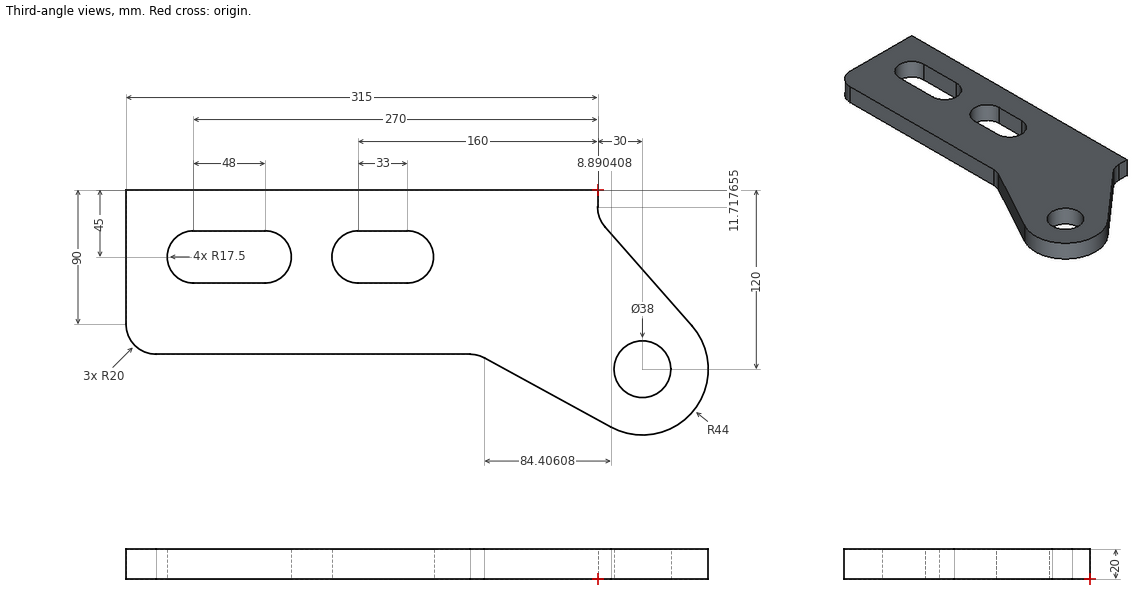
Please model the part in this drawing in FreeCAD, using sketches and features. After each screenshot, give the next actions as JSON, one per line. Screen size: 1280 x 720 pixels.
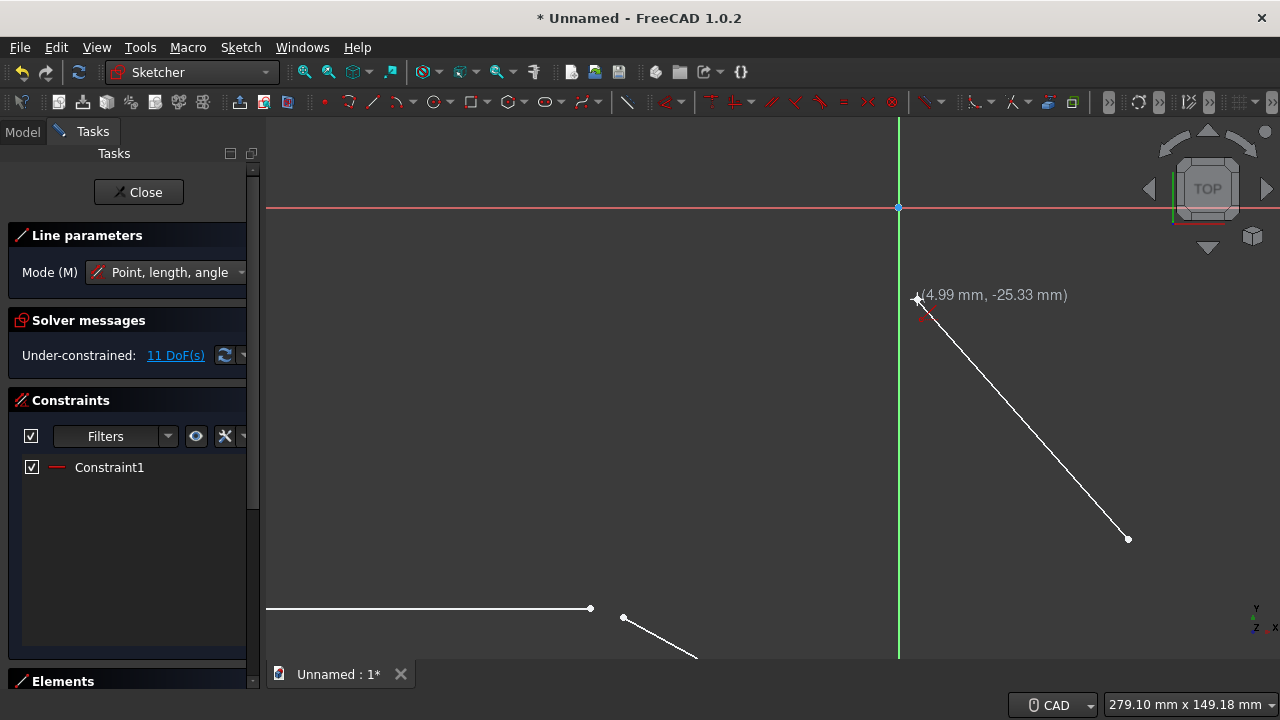
{"action": "left_click", "coordinate": [350, 102]}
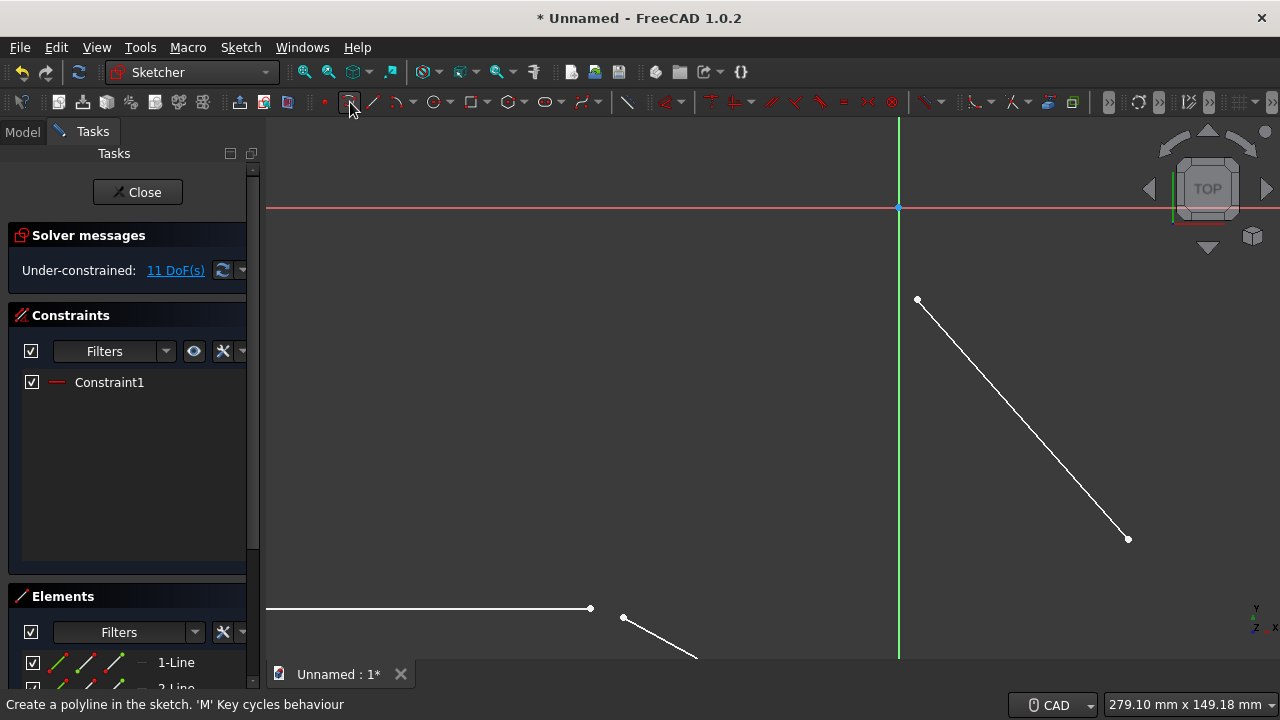
{"action": "left_click", "coordinate": [899, 251]}
{"action": "left_click", "coordinate": [899, 208]}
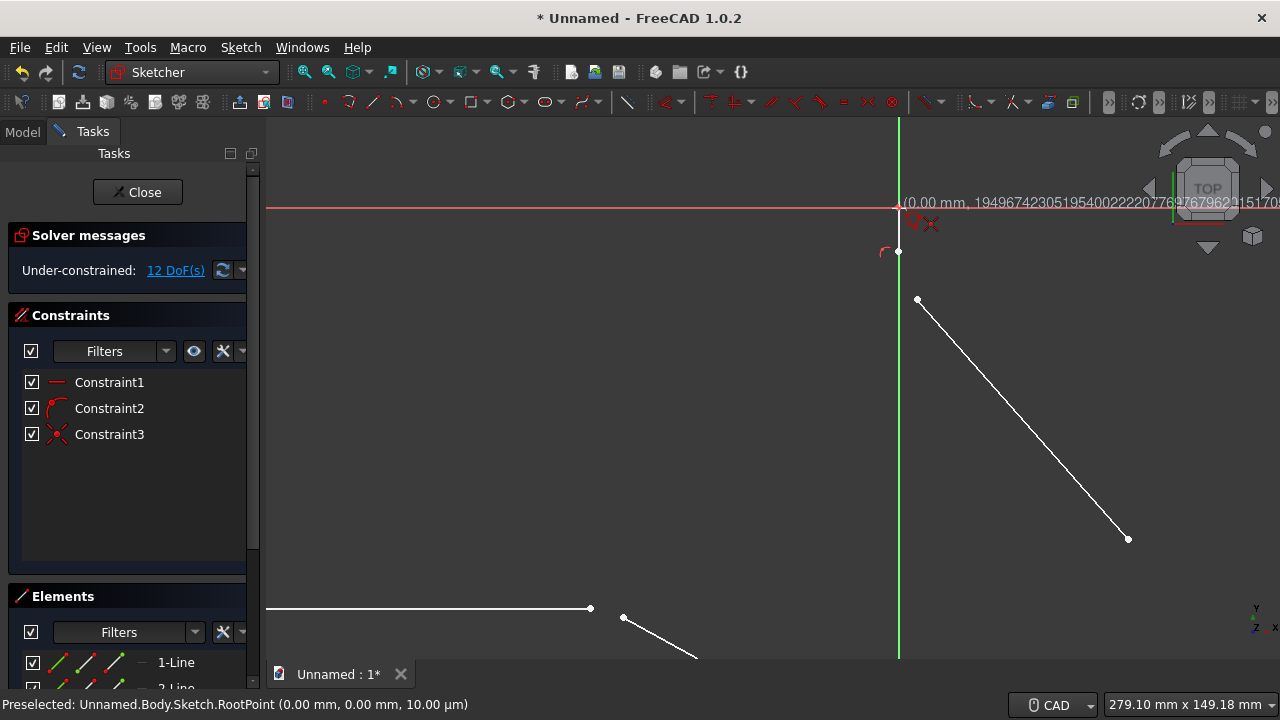
{"action": "scroll", "coordinate": [917, 300], "scroll_direction": "down", "scroll_amount": 4}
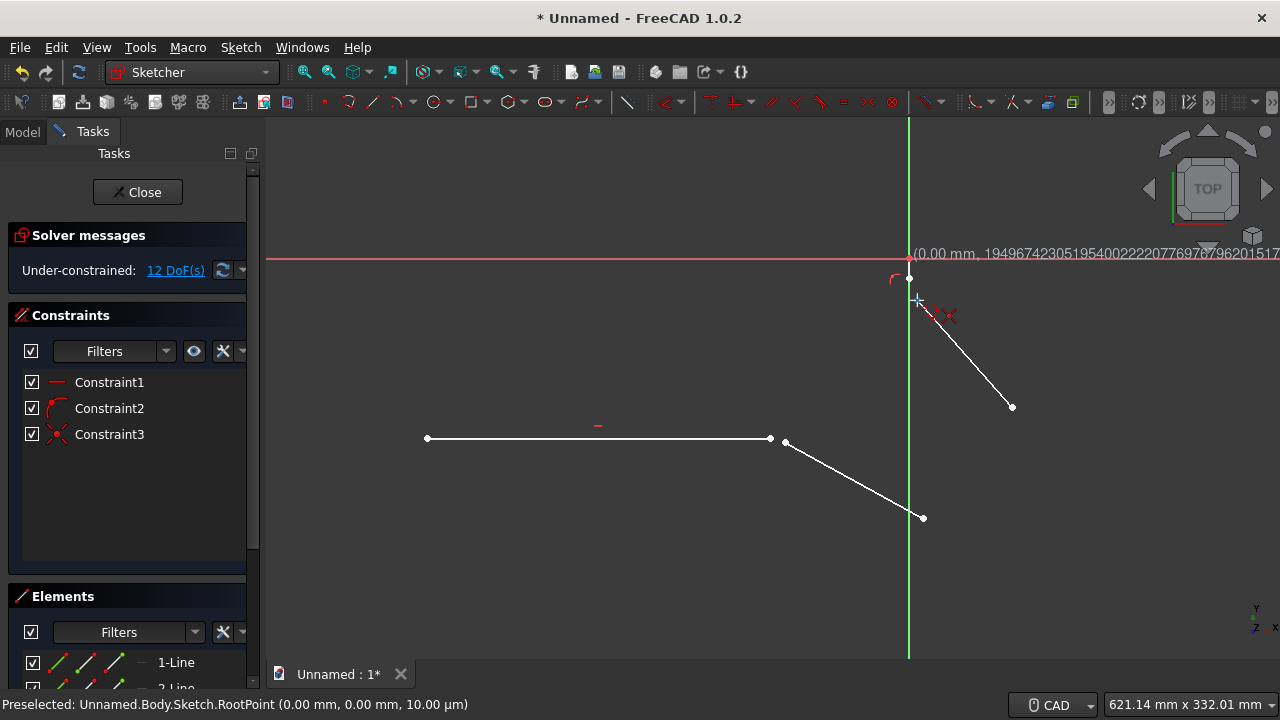
{"action": "left_click", "coordinate": [395, 268]}
{"action": "left_click", "coordinate": [395, 406]}
{"action": "right_click", "coordinate": [395, 406]}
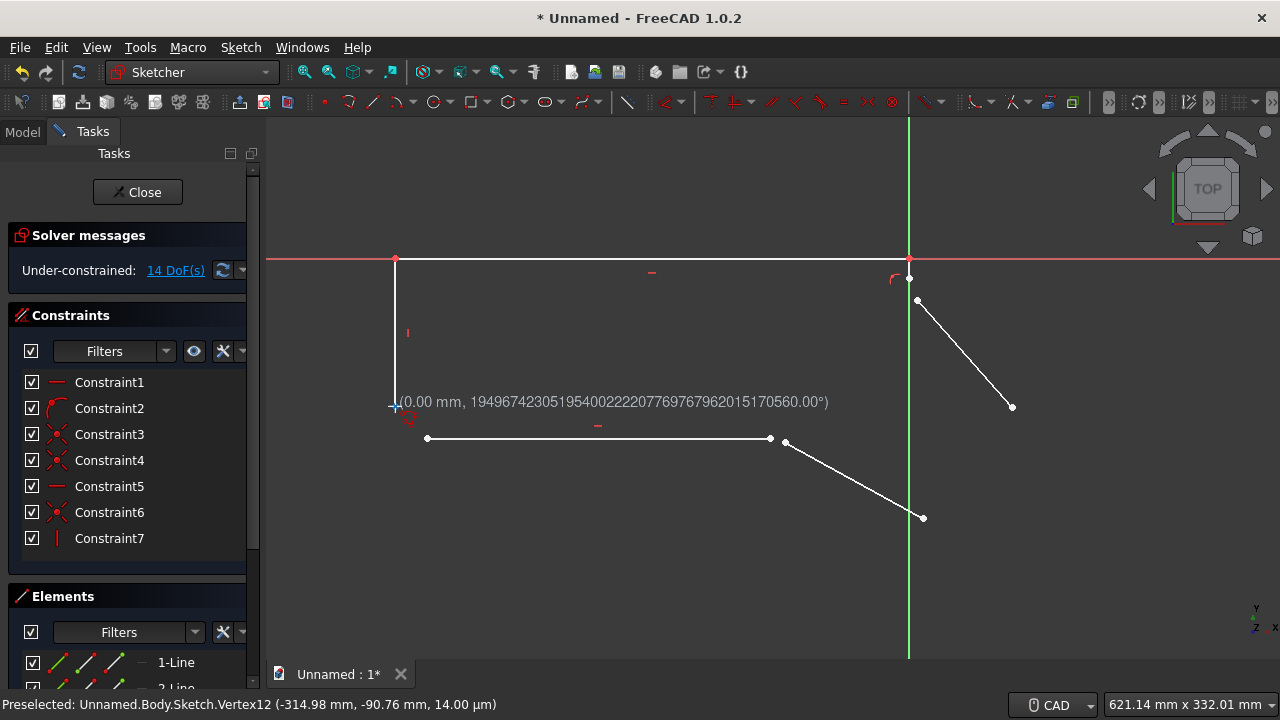
{"action": "left_click", "coordinate": [416, 102]}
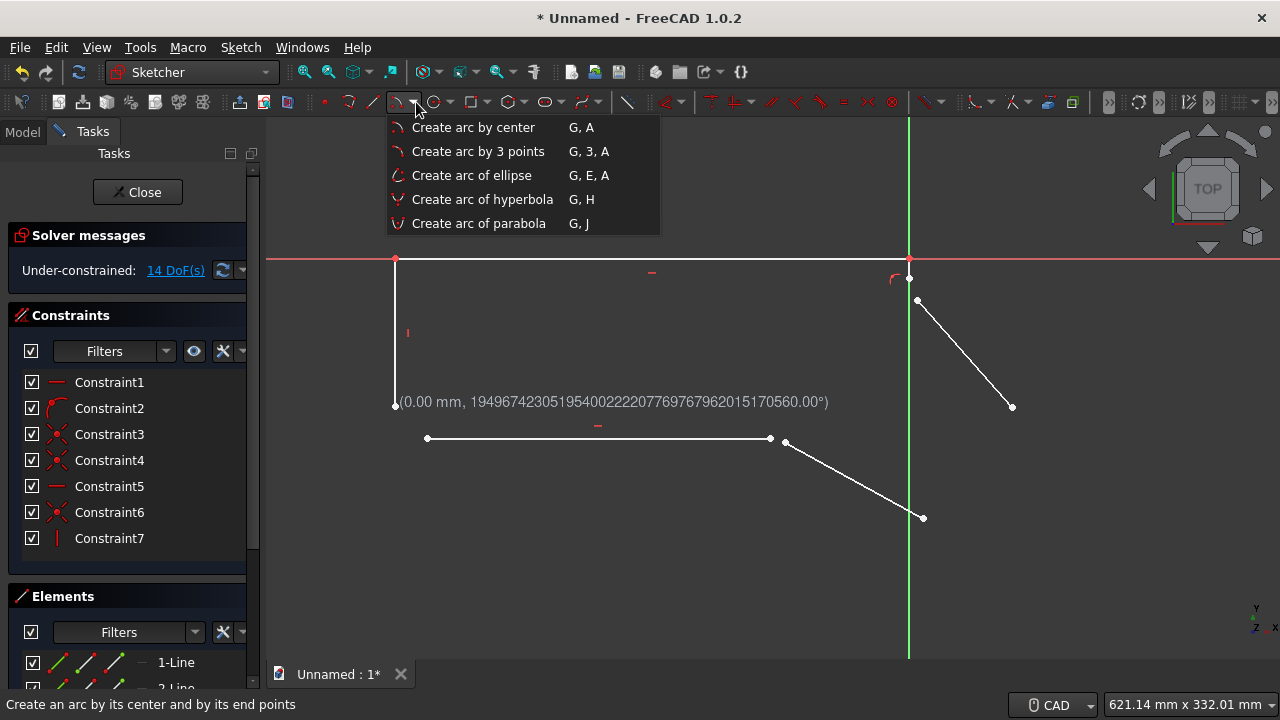
{"action": "left_click", "coordinate": [524, 151]}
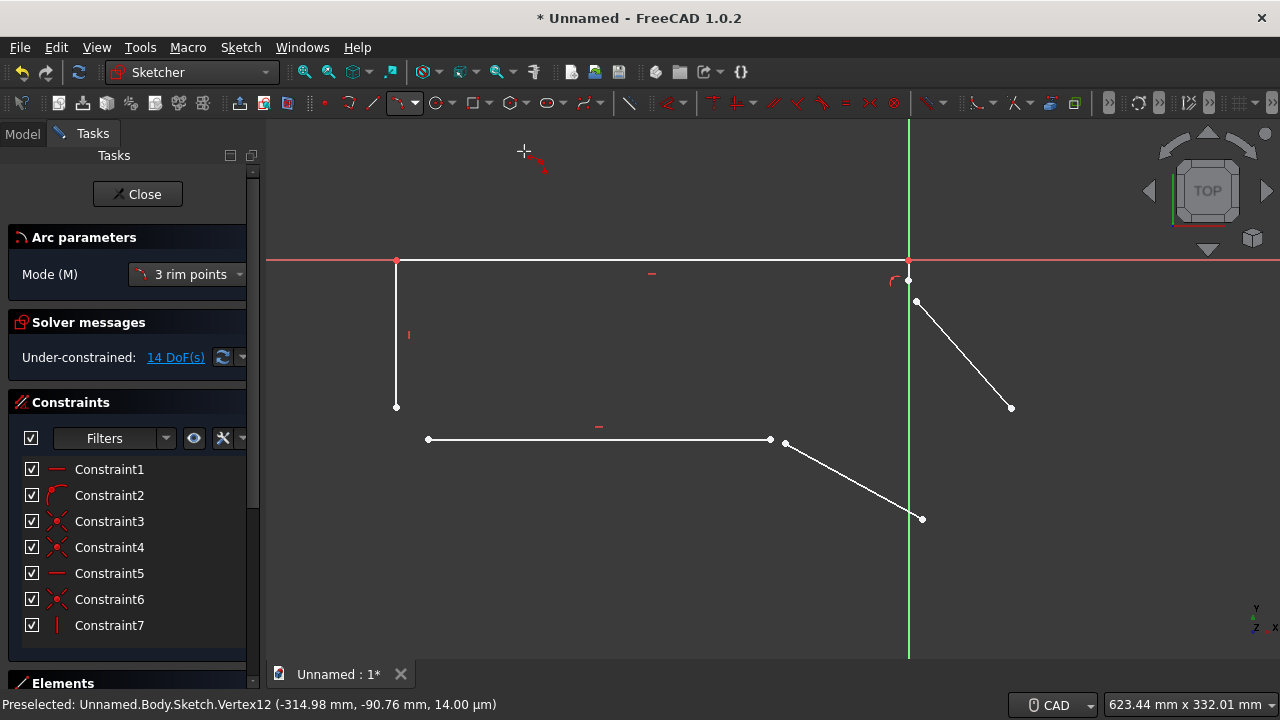
{"action": "left_click", "coordinate": [770, 440]}
{"action": "left_click", "coordinate": [785, 444]}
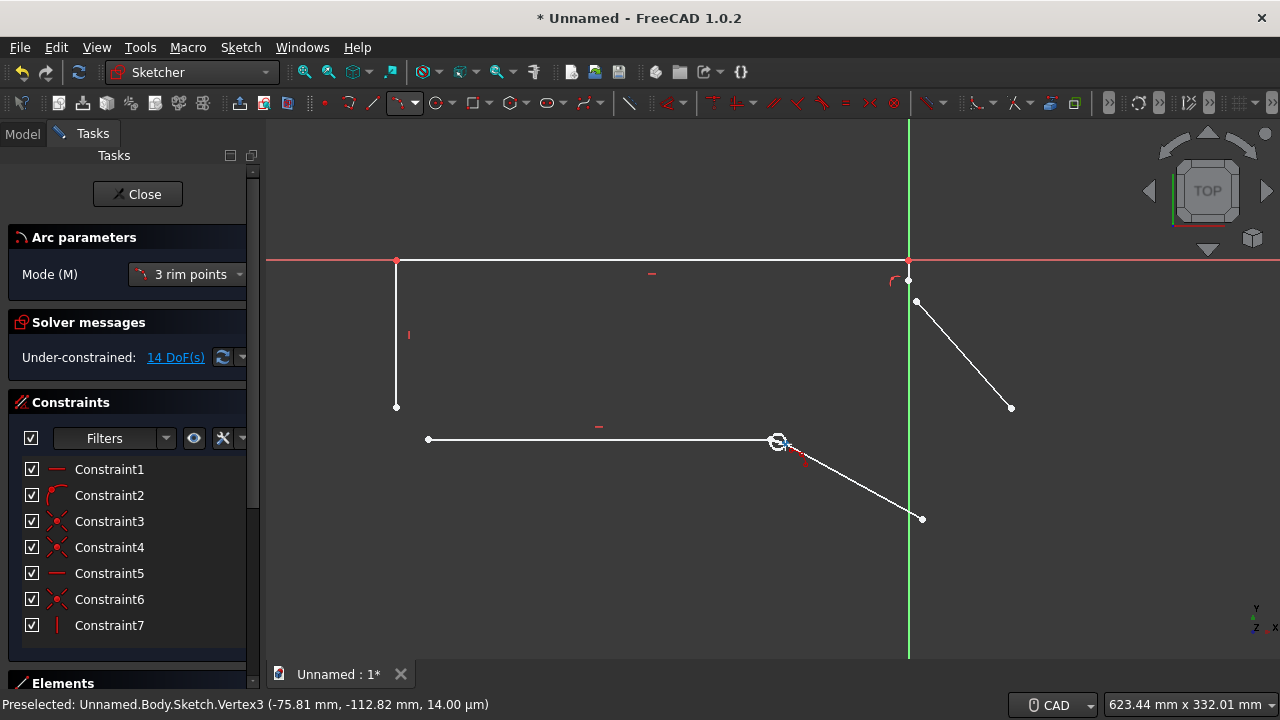
{"action": "scroll", "coordinate": [778, 440], "scroll_direction": "up", "scroll_amount": 14}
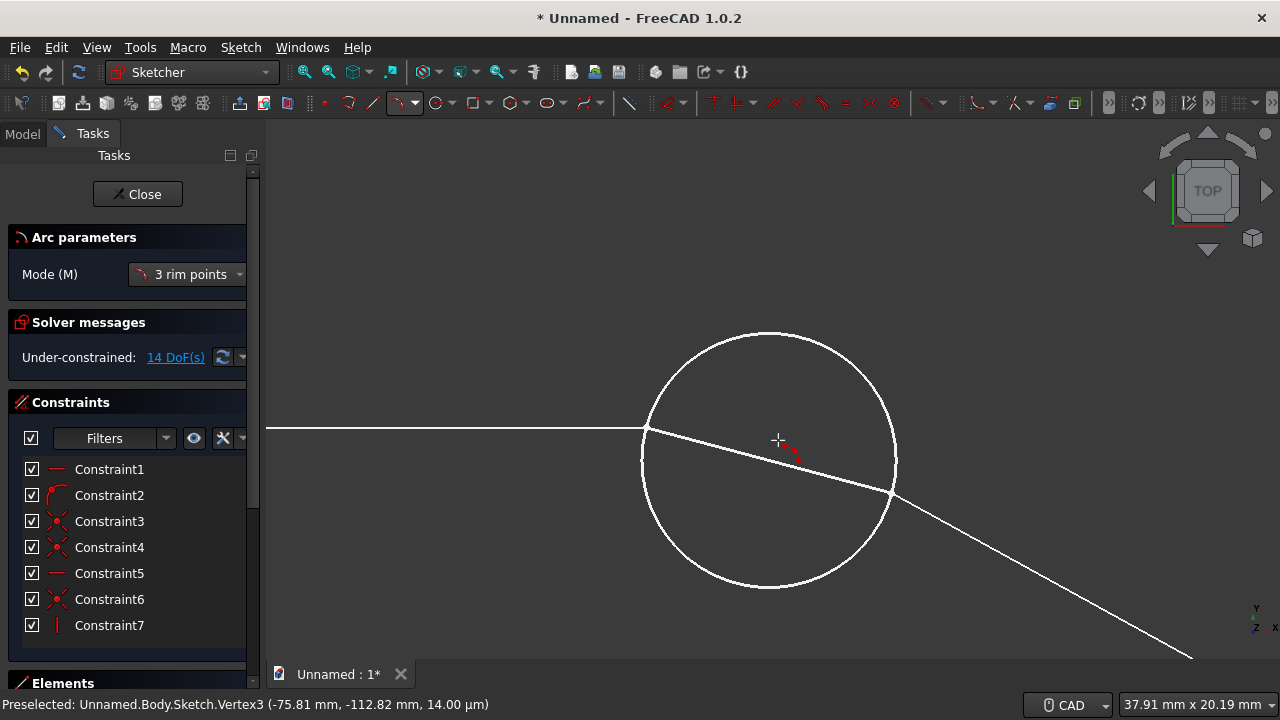
{"action": "left_click", "coordinate": [776, 435]}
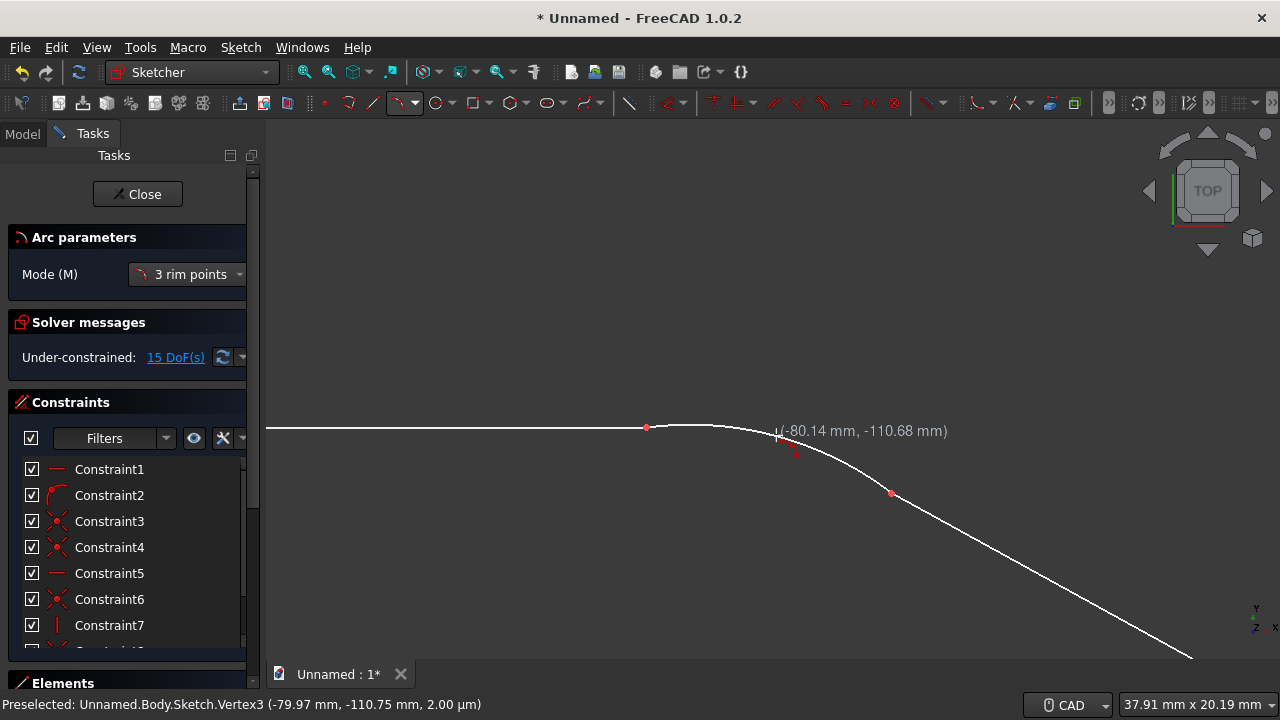
{"action": "scroll", "coordinate": [778, 440], "scroll_direction": "down", "scroll_amount": 14}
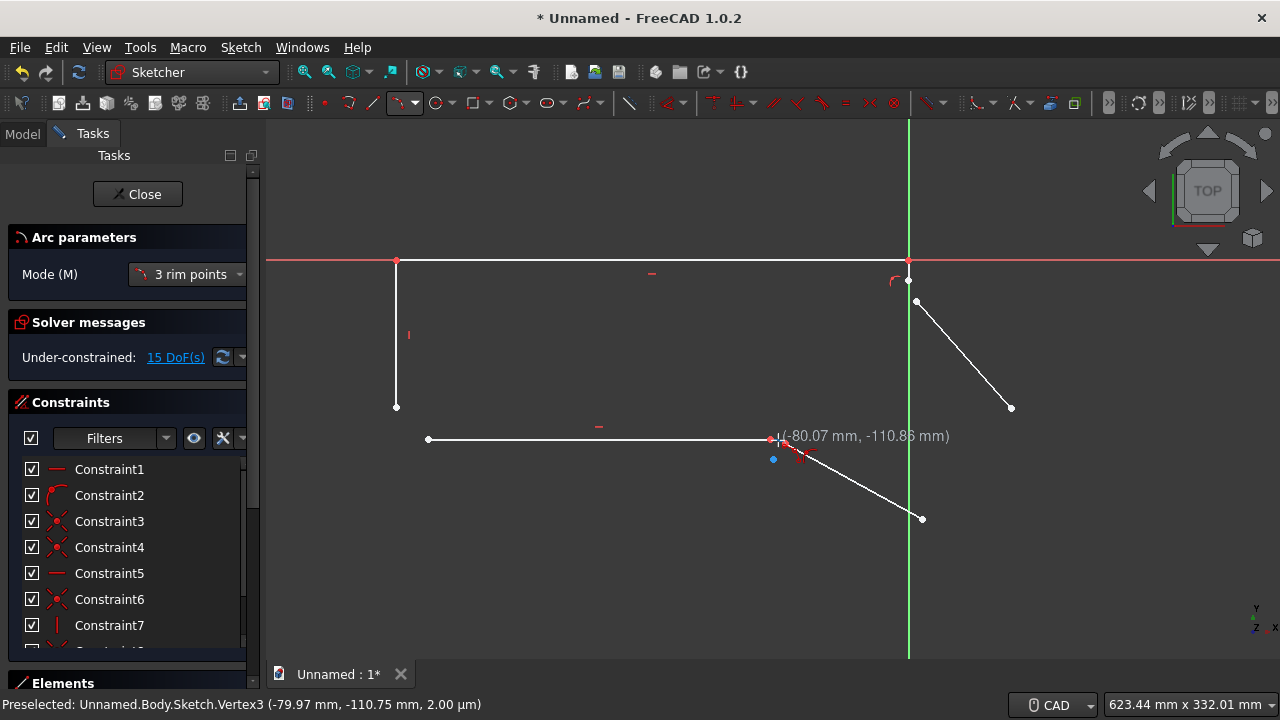
{"action": "left_click", "coordinate": [923, 520]}
{"action": "left_click", "coordinate": [1012, 409]}
{"action": "left_click", "coordinate": [1013, 500]}